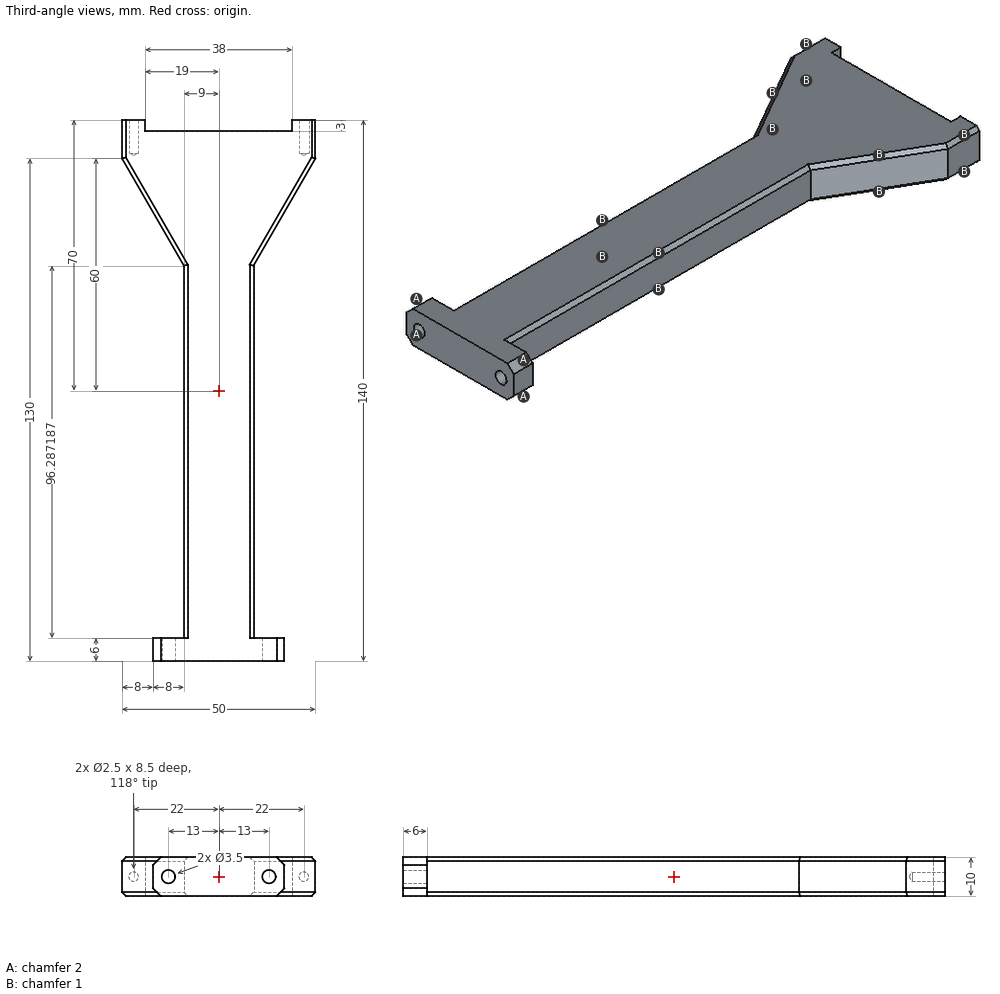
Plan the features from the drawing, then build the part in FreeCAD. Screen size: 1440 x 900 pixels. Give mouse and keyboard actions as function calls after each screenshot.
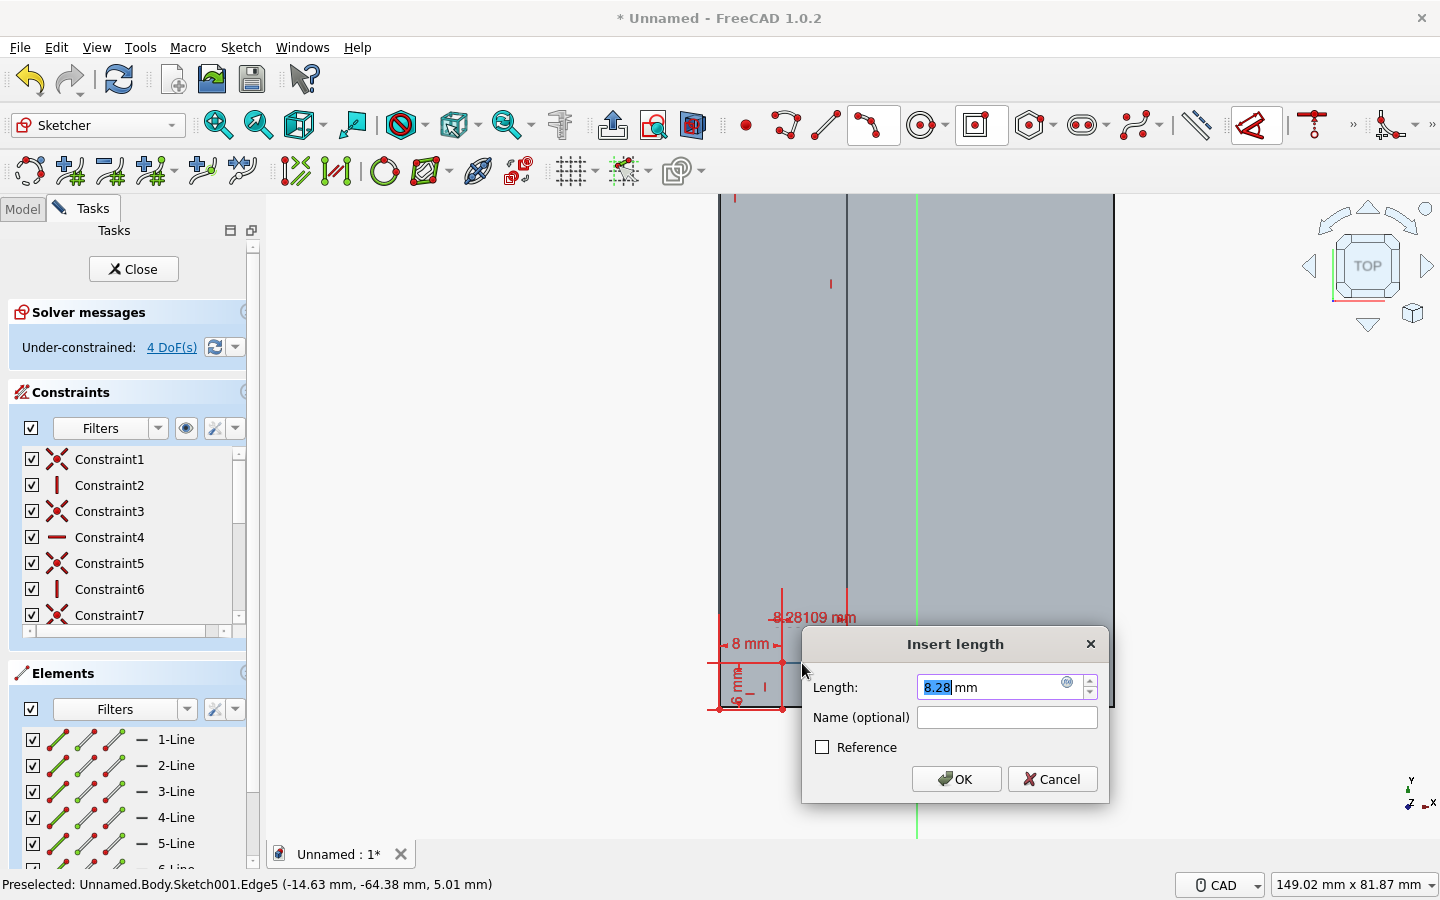
text(8)
key(Return)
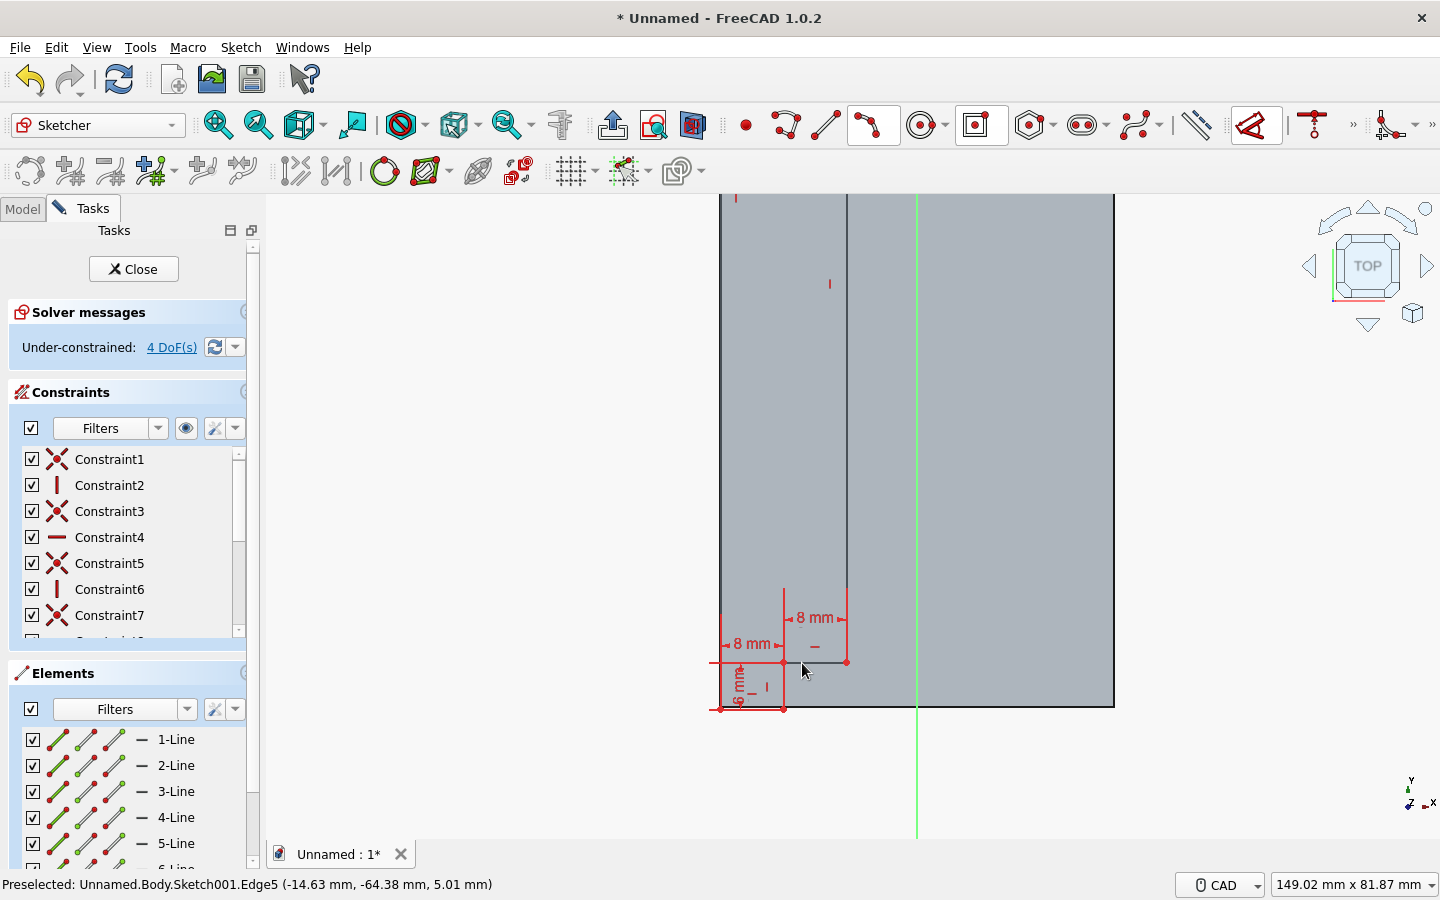
scroll(765, 704, down, 5)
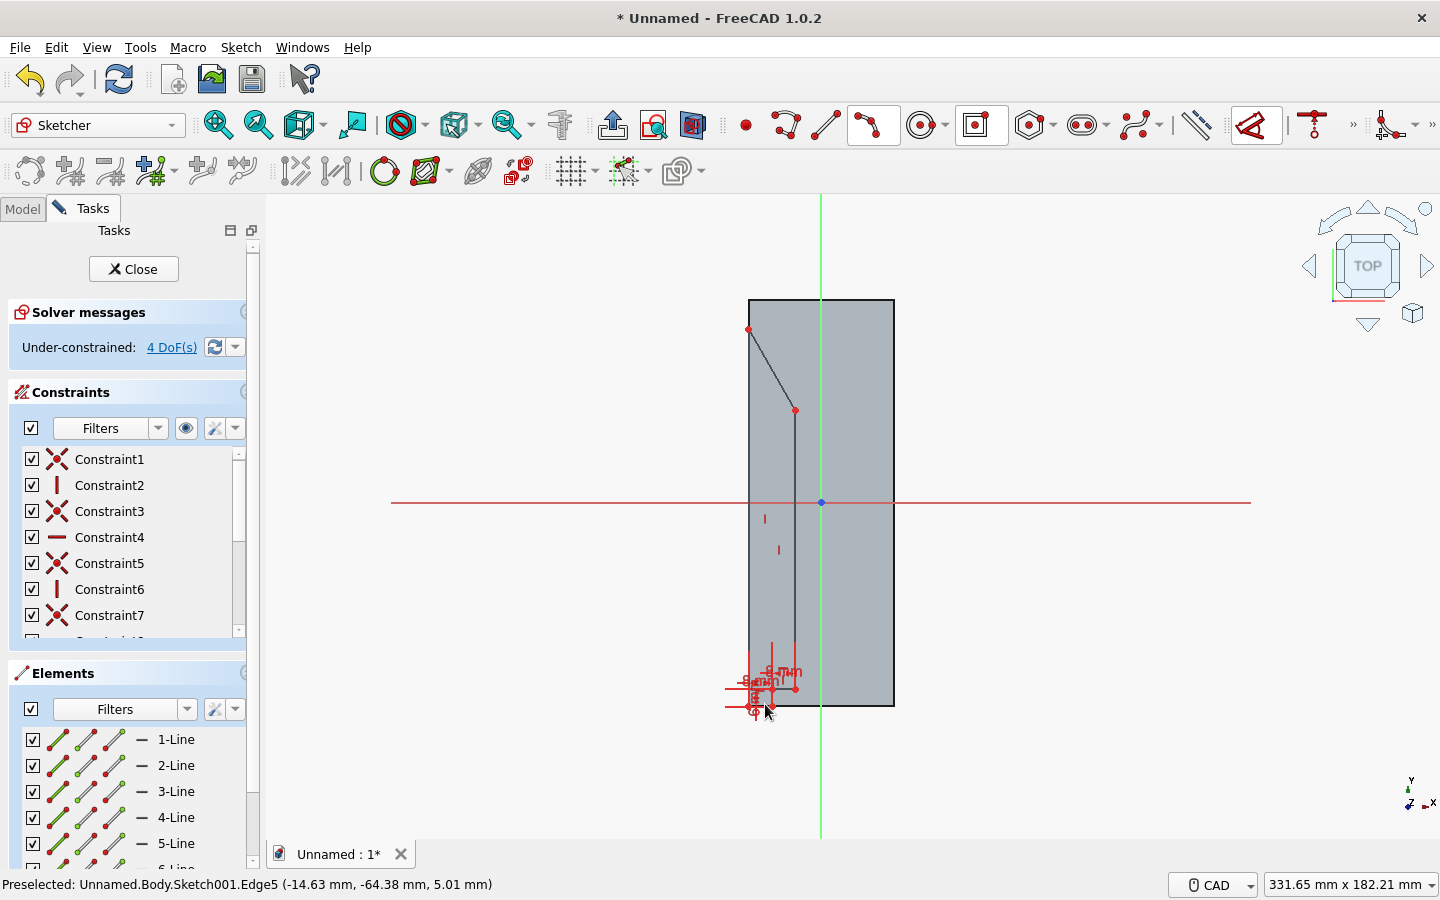
scroll(795, 411, up, 3)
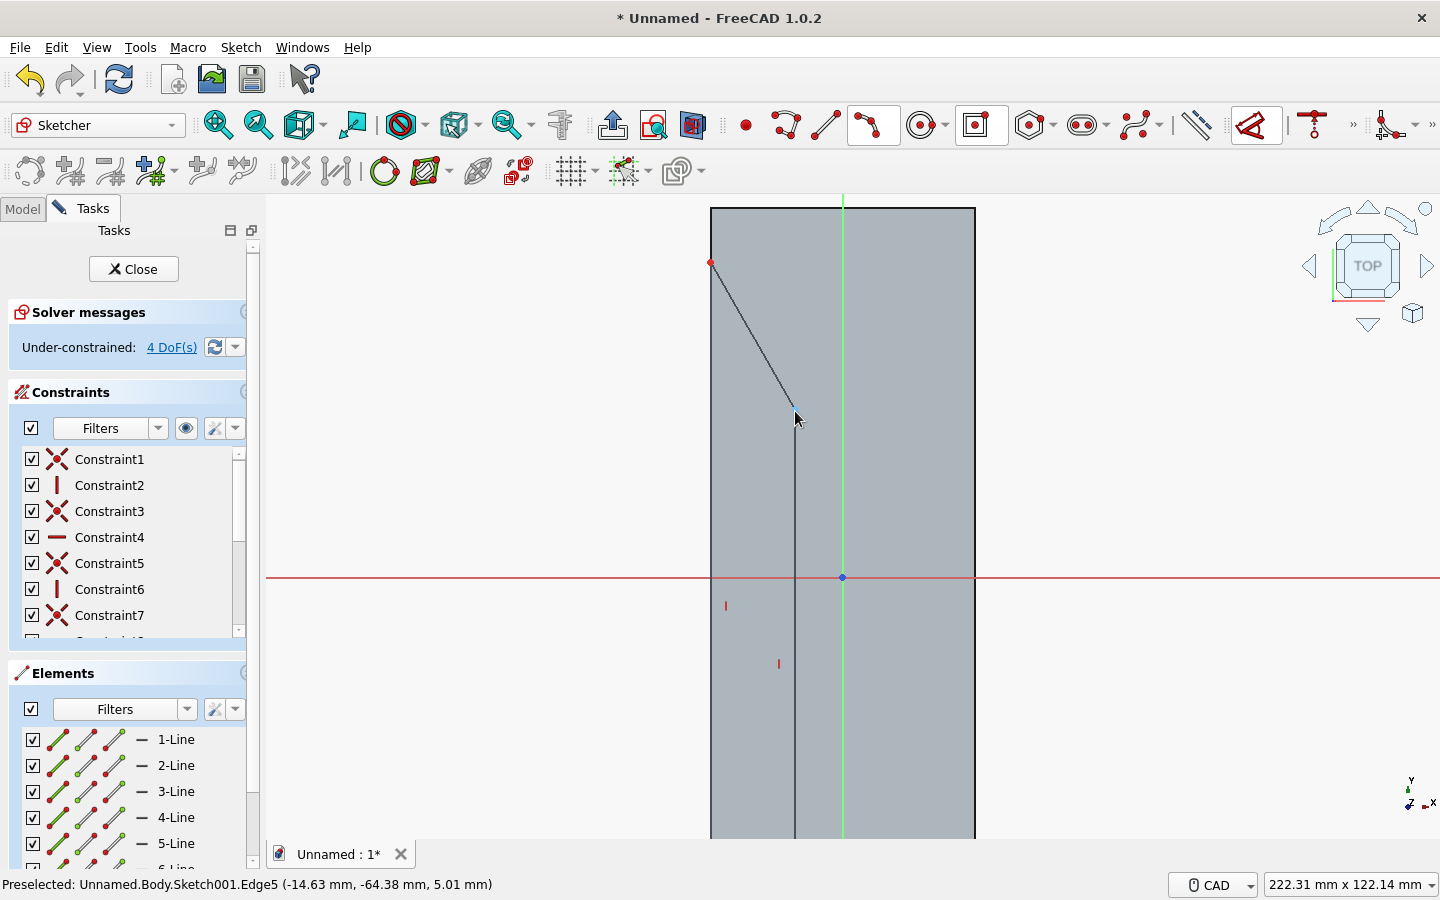
click(795, 410)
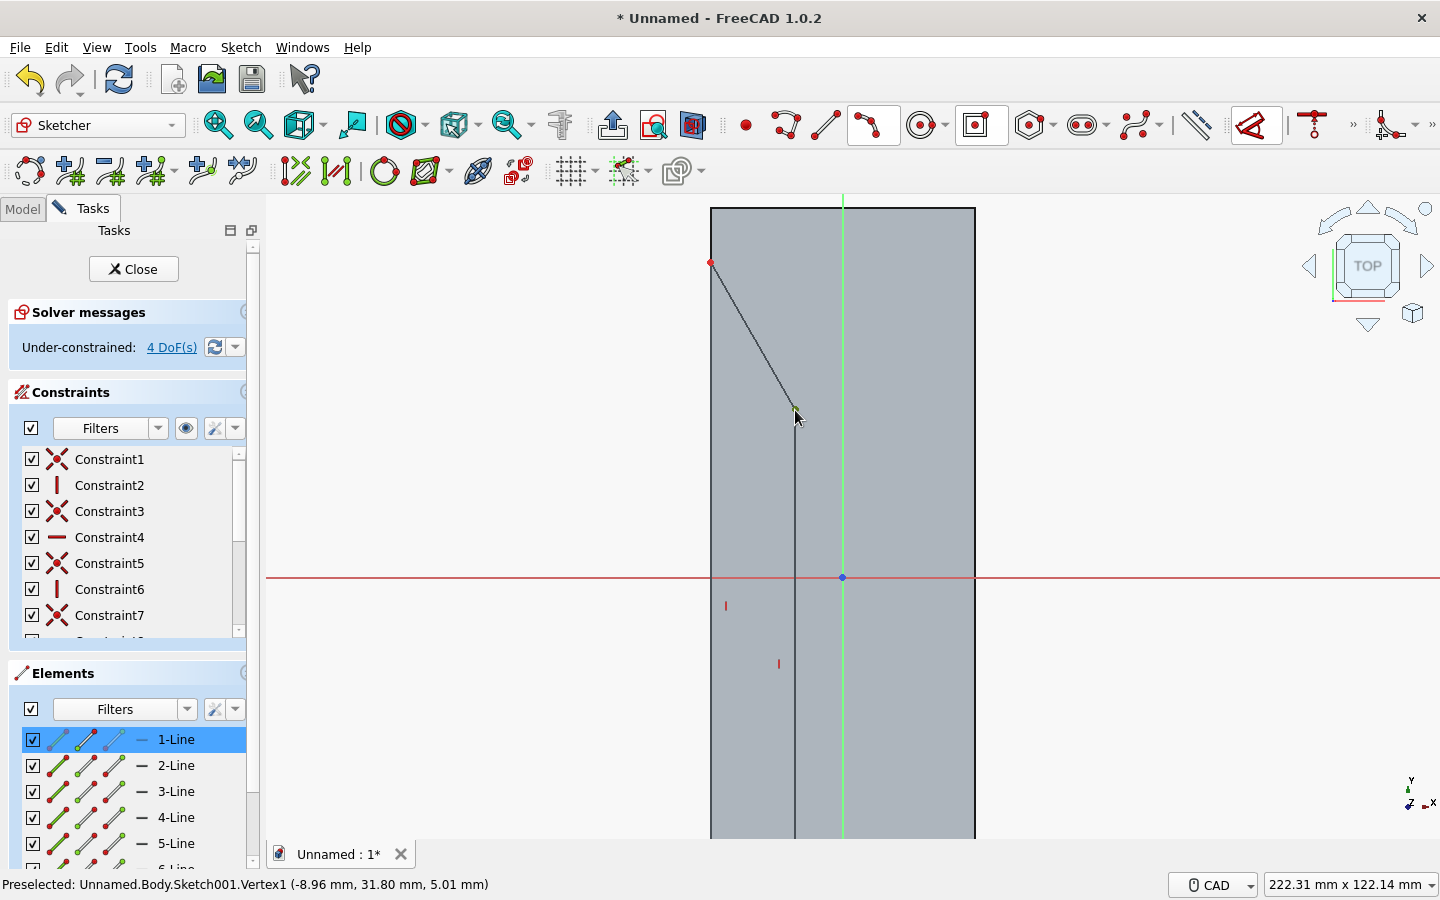
click(1276, 126)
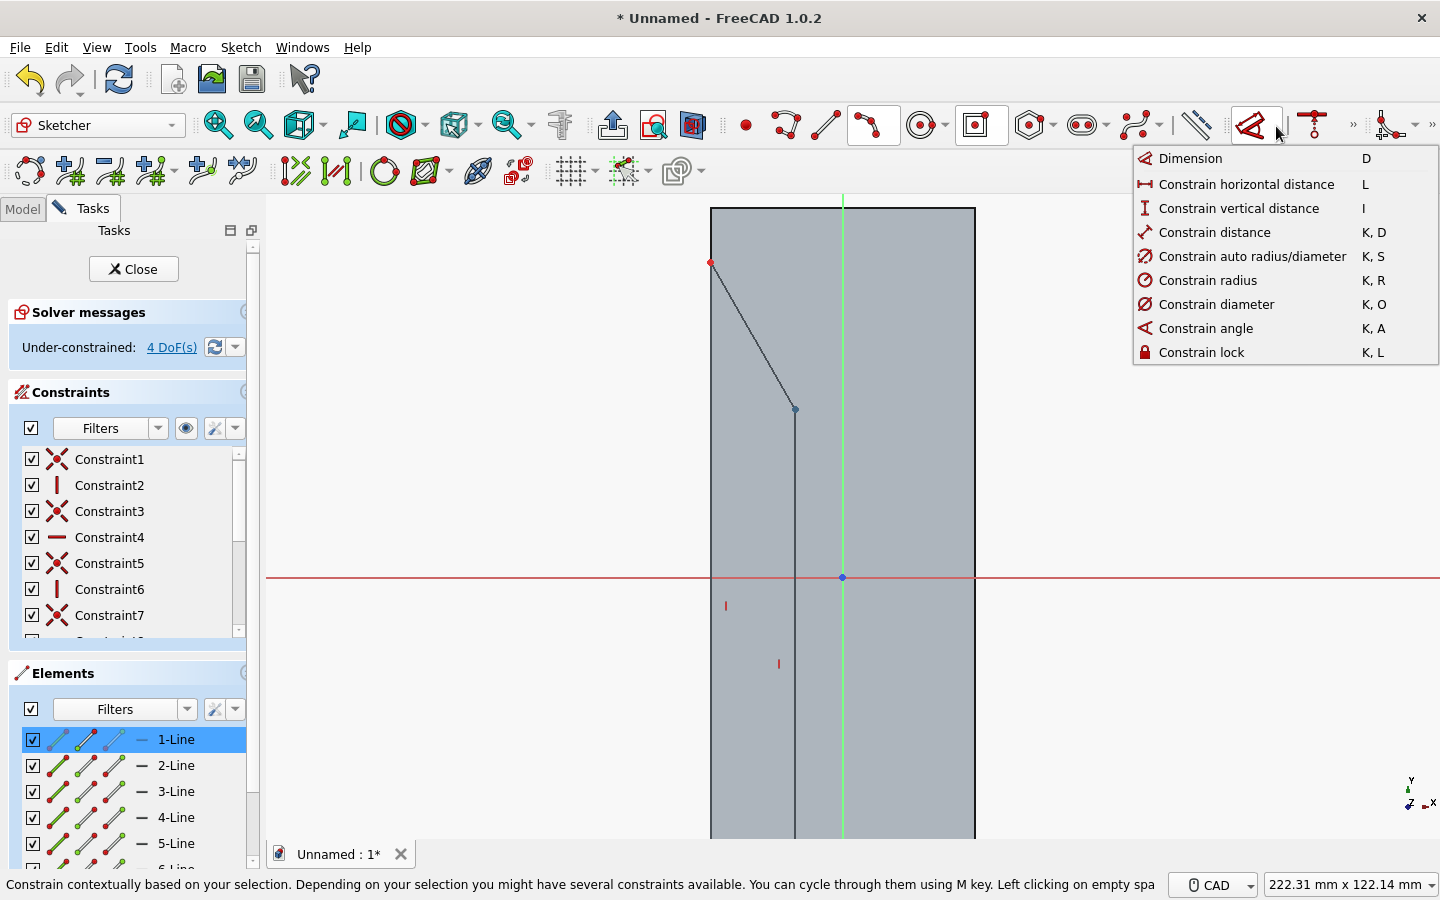
click(1286, 184)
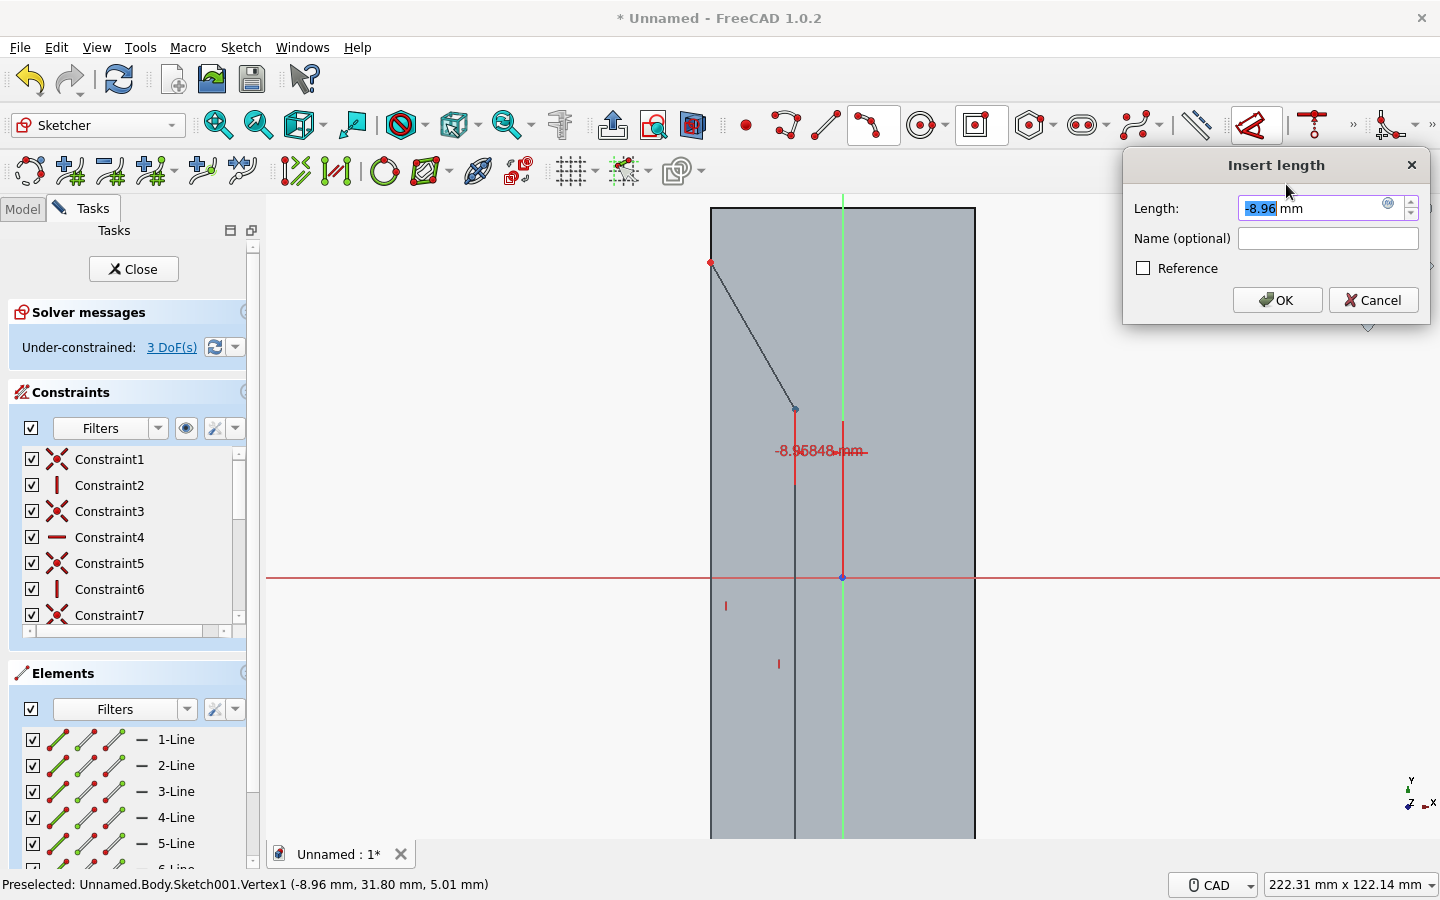
text(-9)
key(Return)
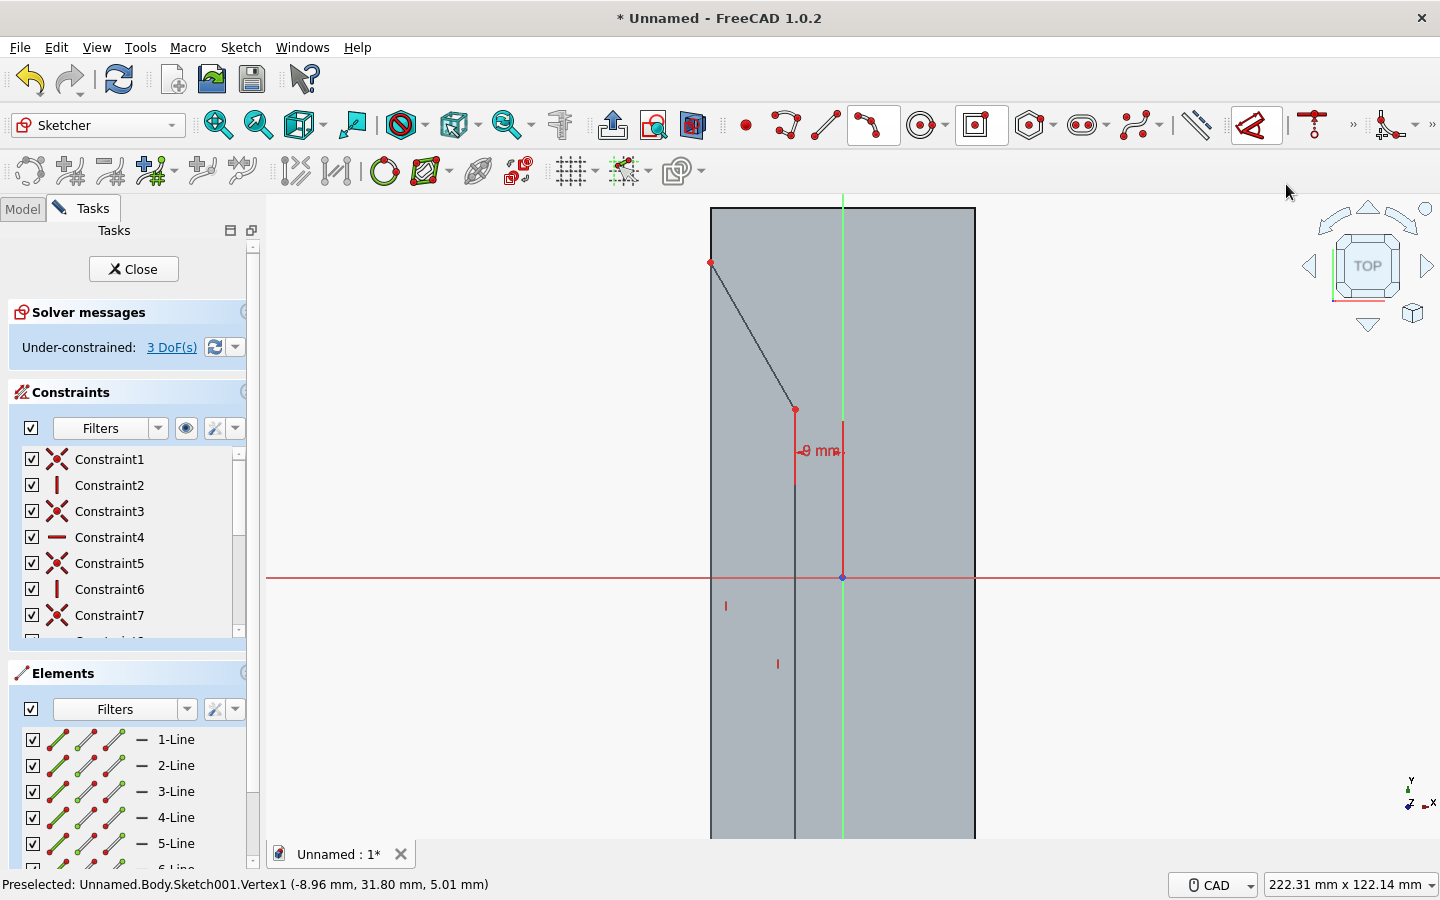
click(711, 468)